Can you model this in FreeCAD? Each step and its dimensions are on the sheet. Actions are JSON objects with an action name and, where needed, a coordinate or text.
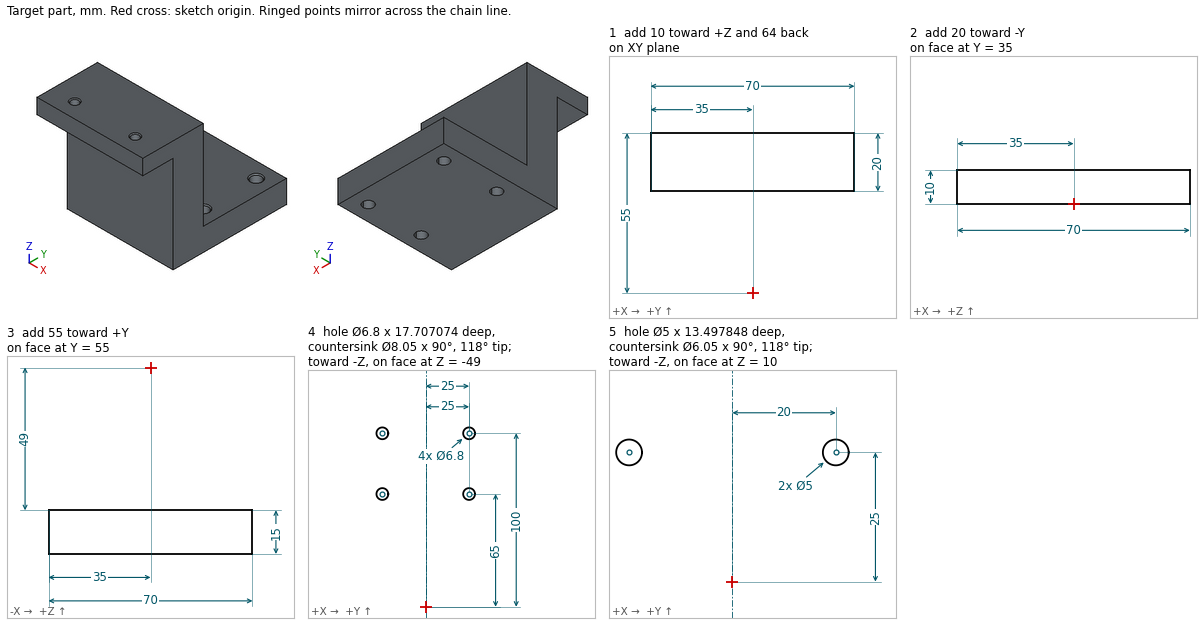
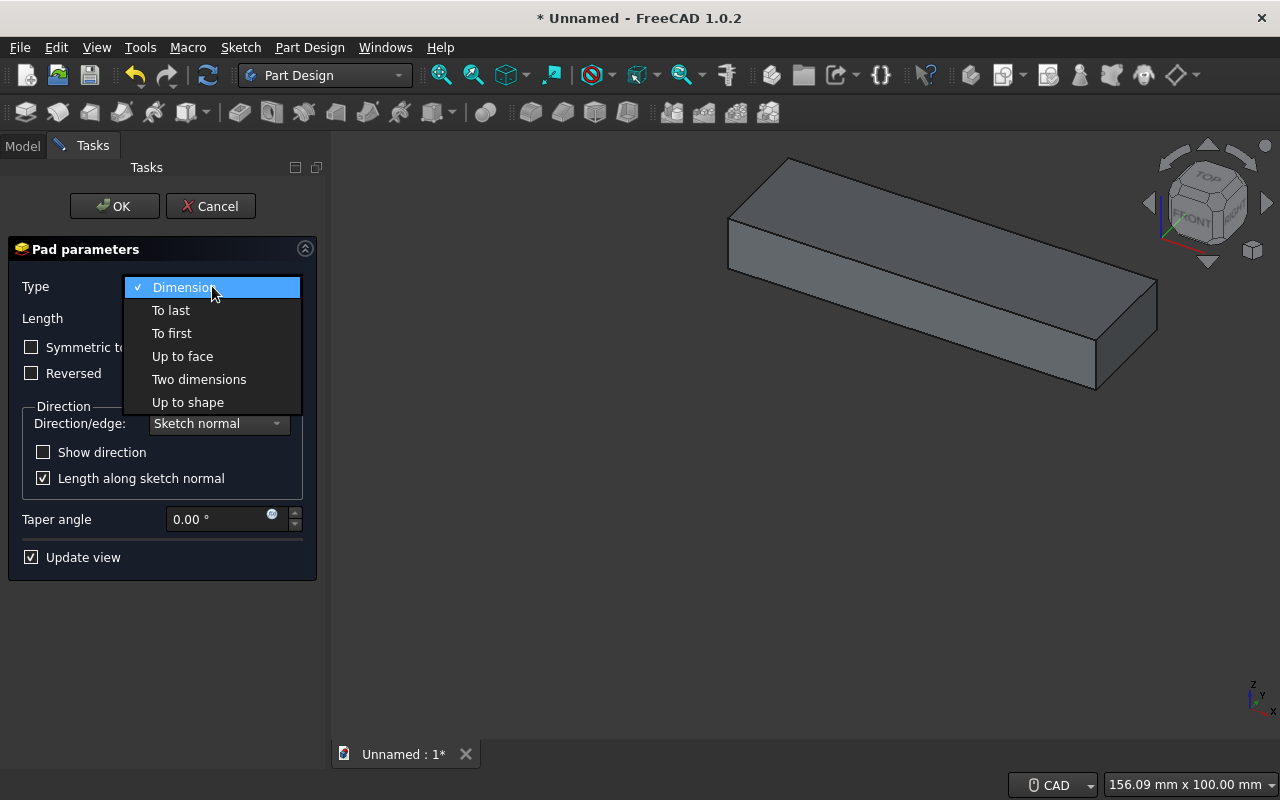
{"action": "left_click", "coordinate": [212, 380]}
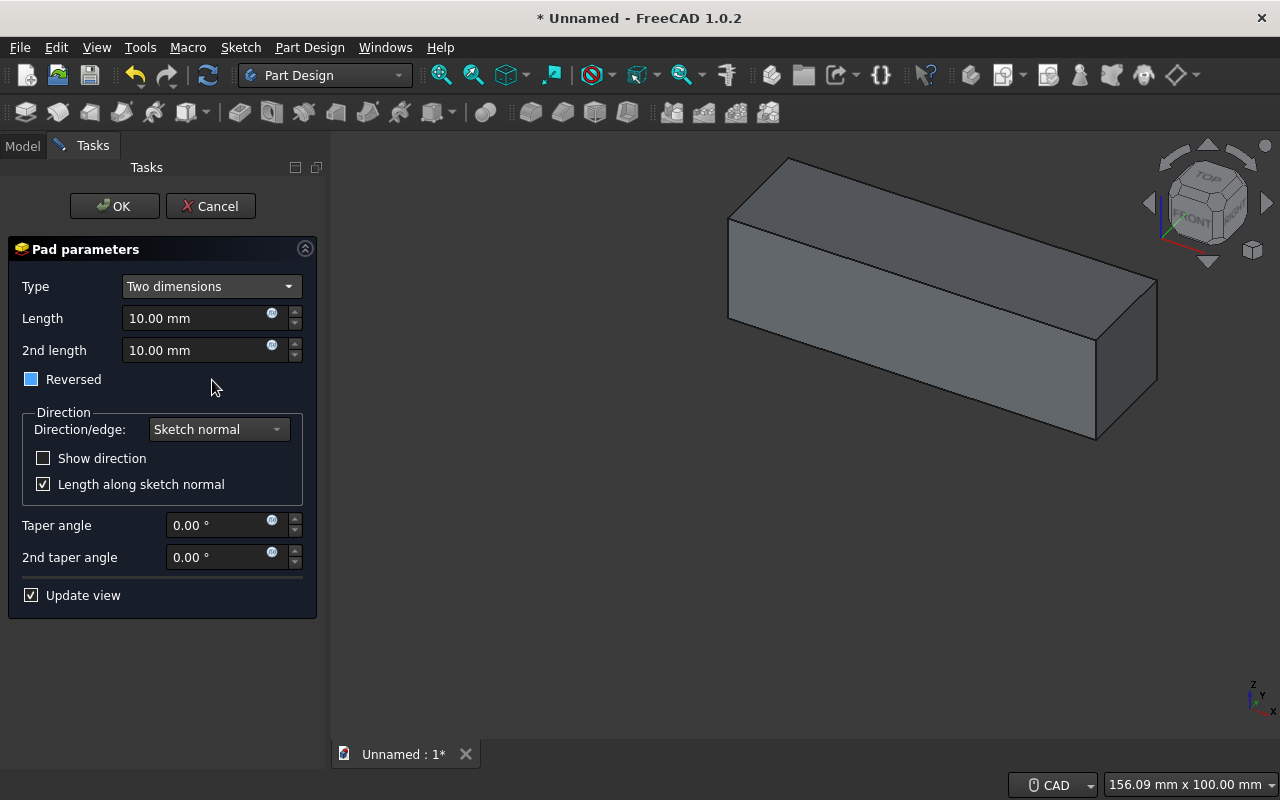
{"action": "triple_click", "coordinate": [204, 318]}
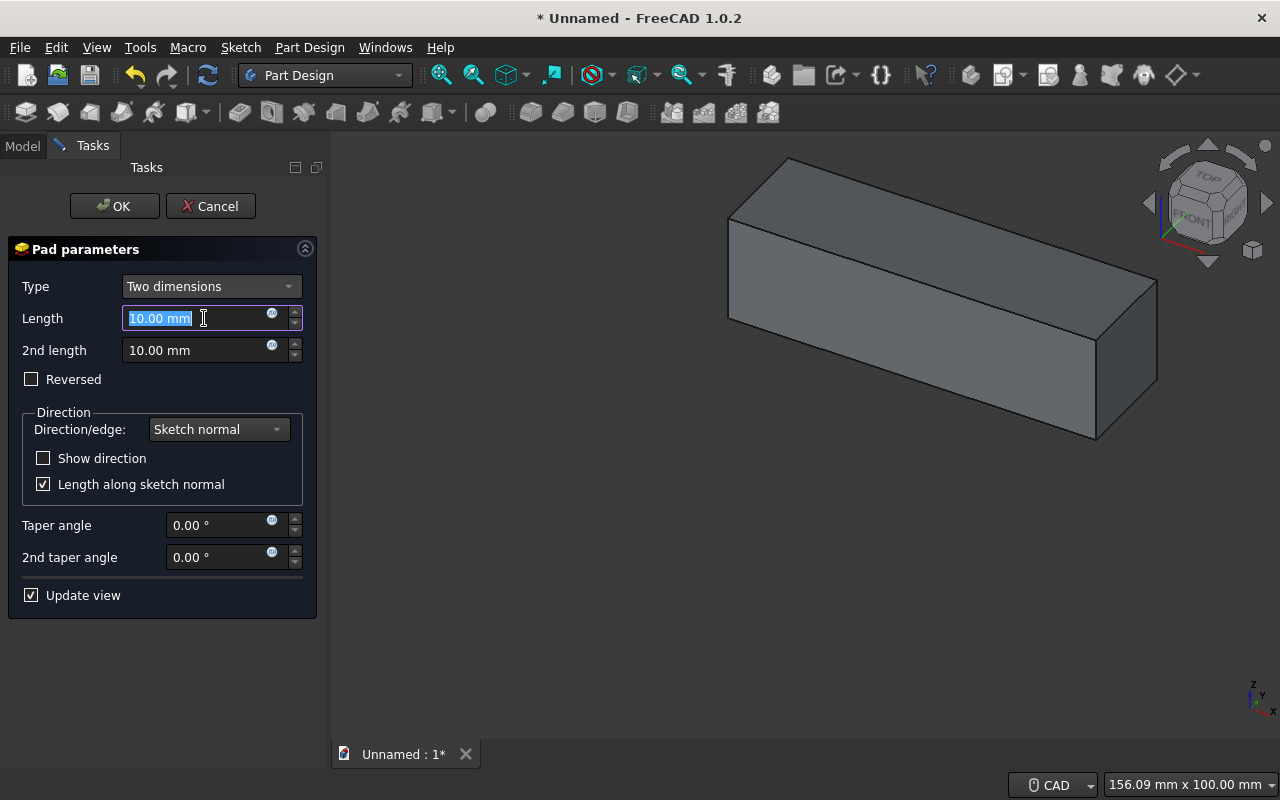
{"action": "type", "text": "10"}
{"action": "key", "text": "Tab"}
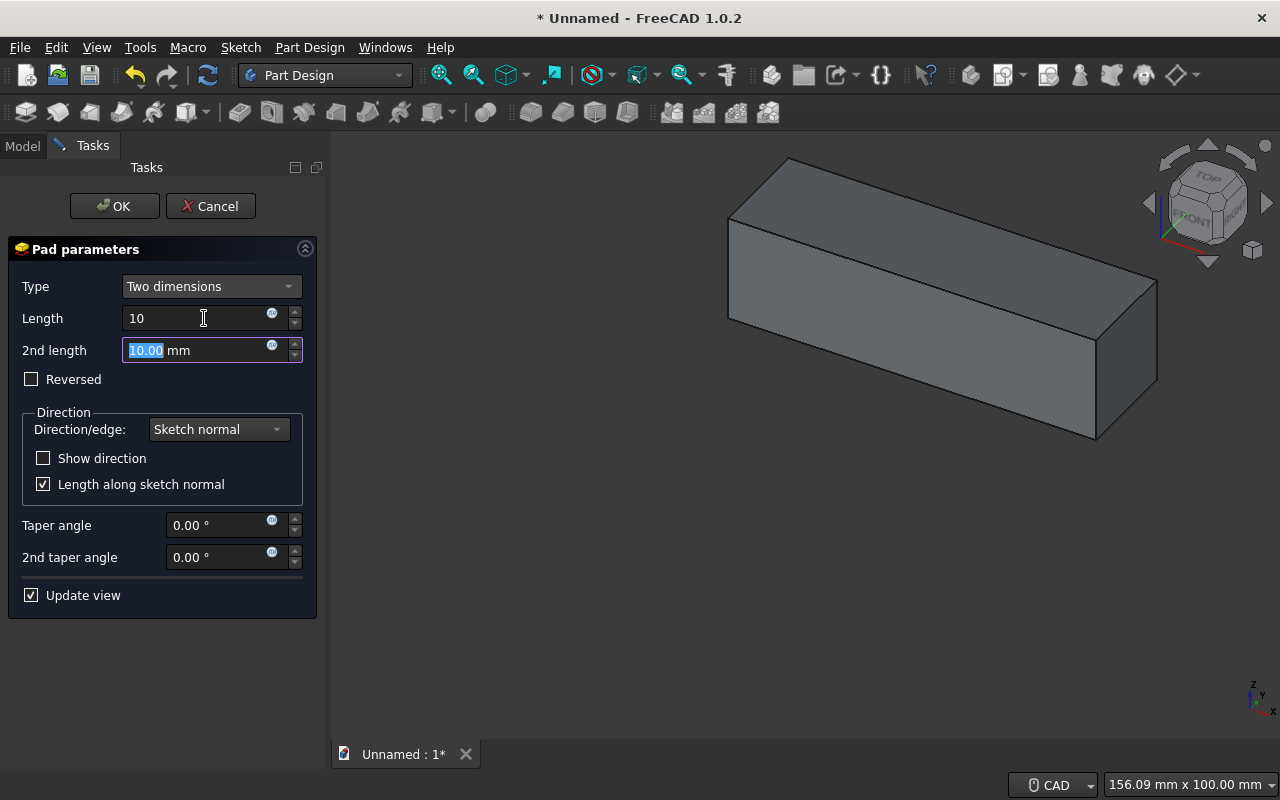
{"action": "type", "text": "64"}
{"action": "key", "text": "Tab"}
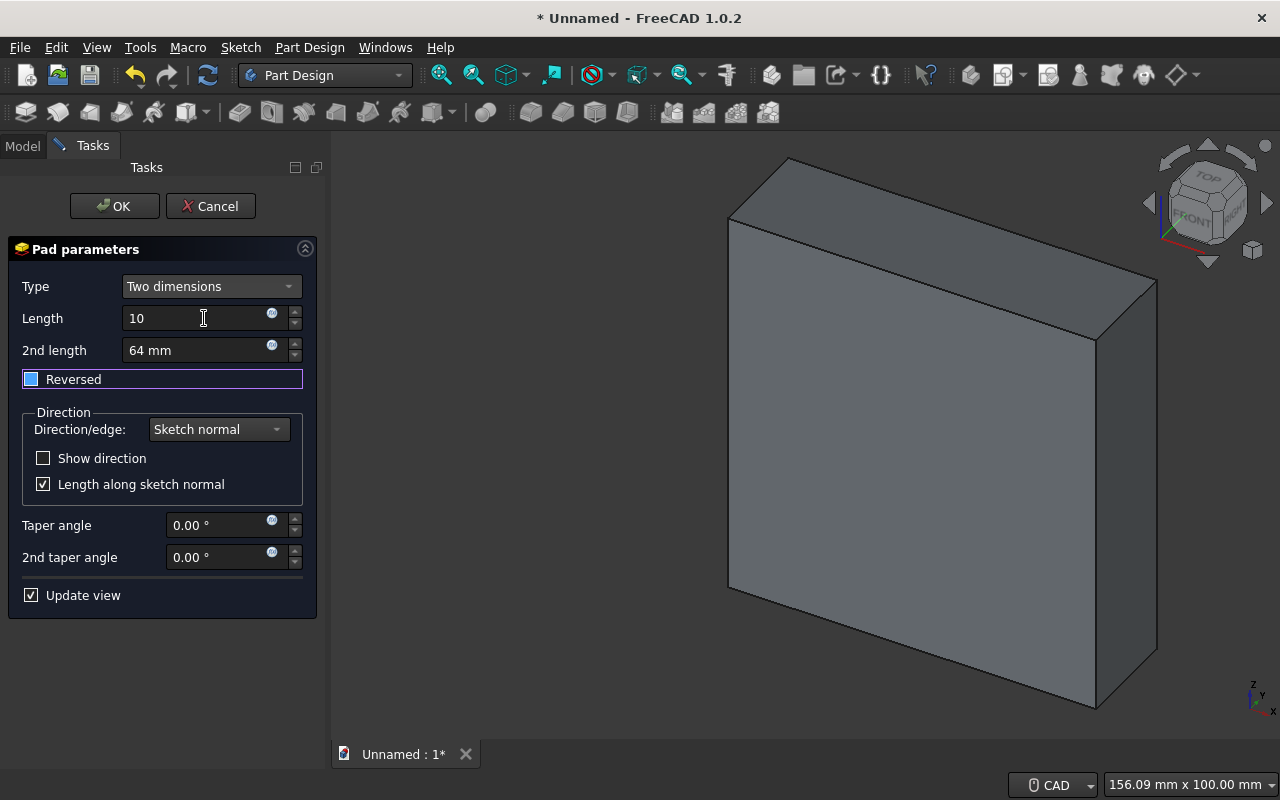
{"action": "left_click", "coordinate": [115, 206]}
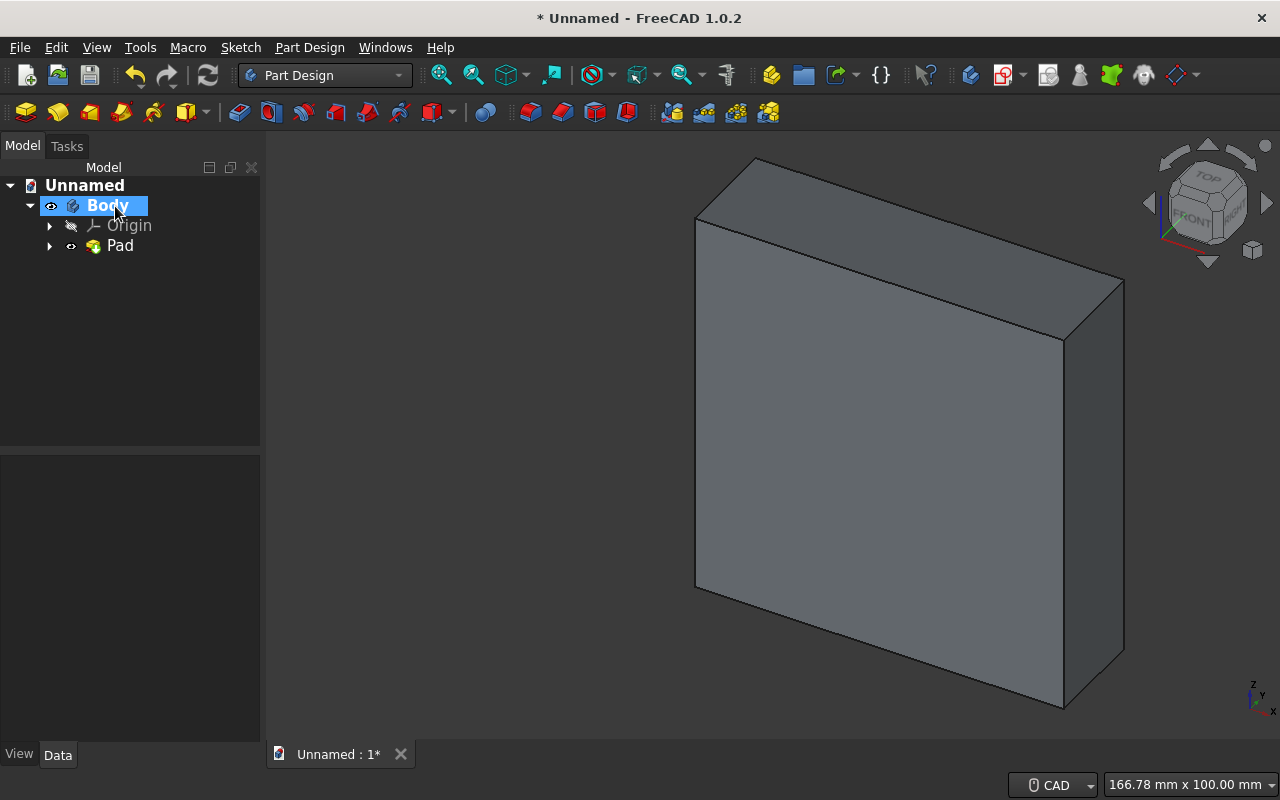
{"action": "left_click", "coordinate": [879, 463]}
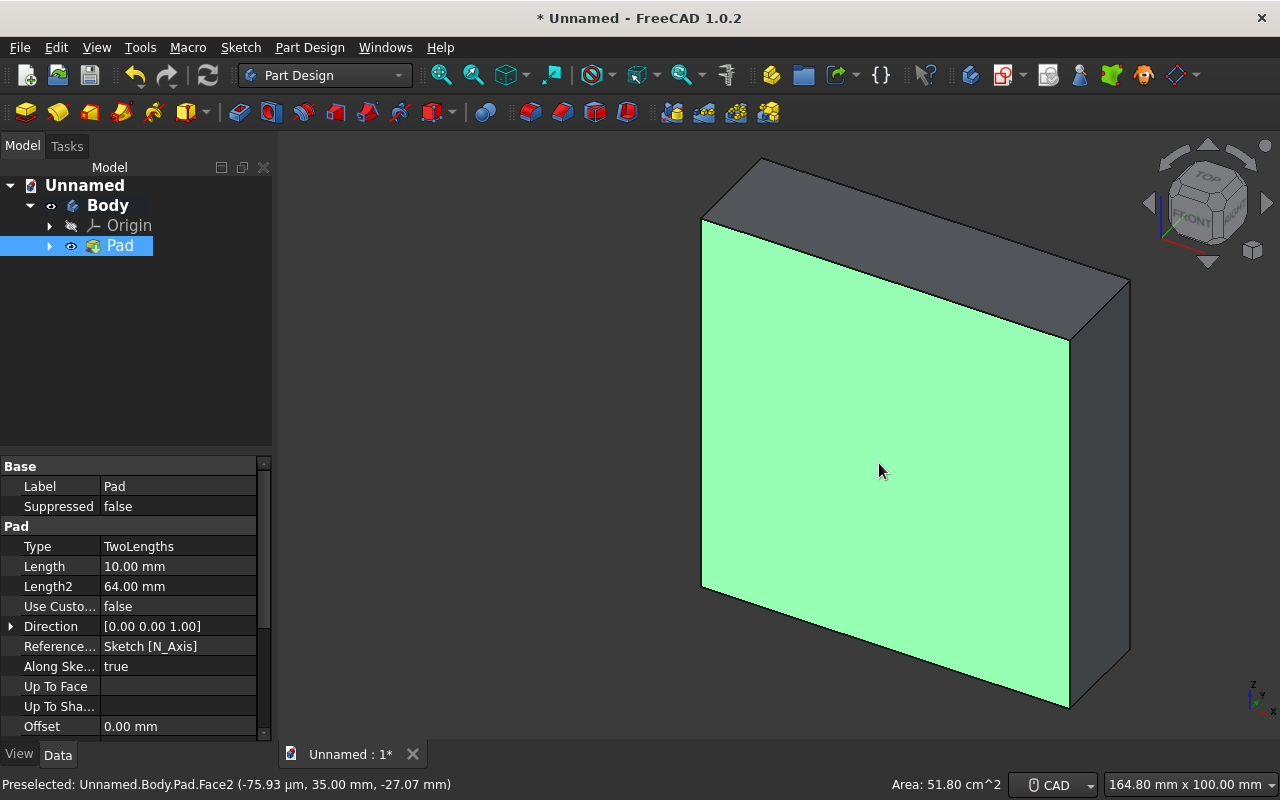
{"action": "left_click", "coordinate": [1004, 76]}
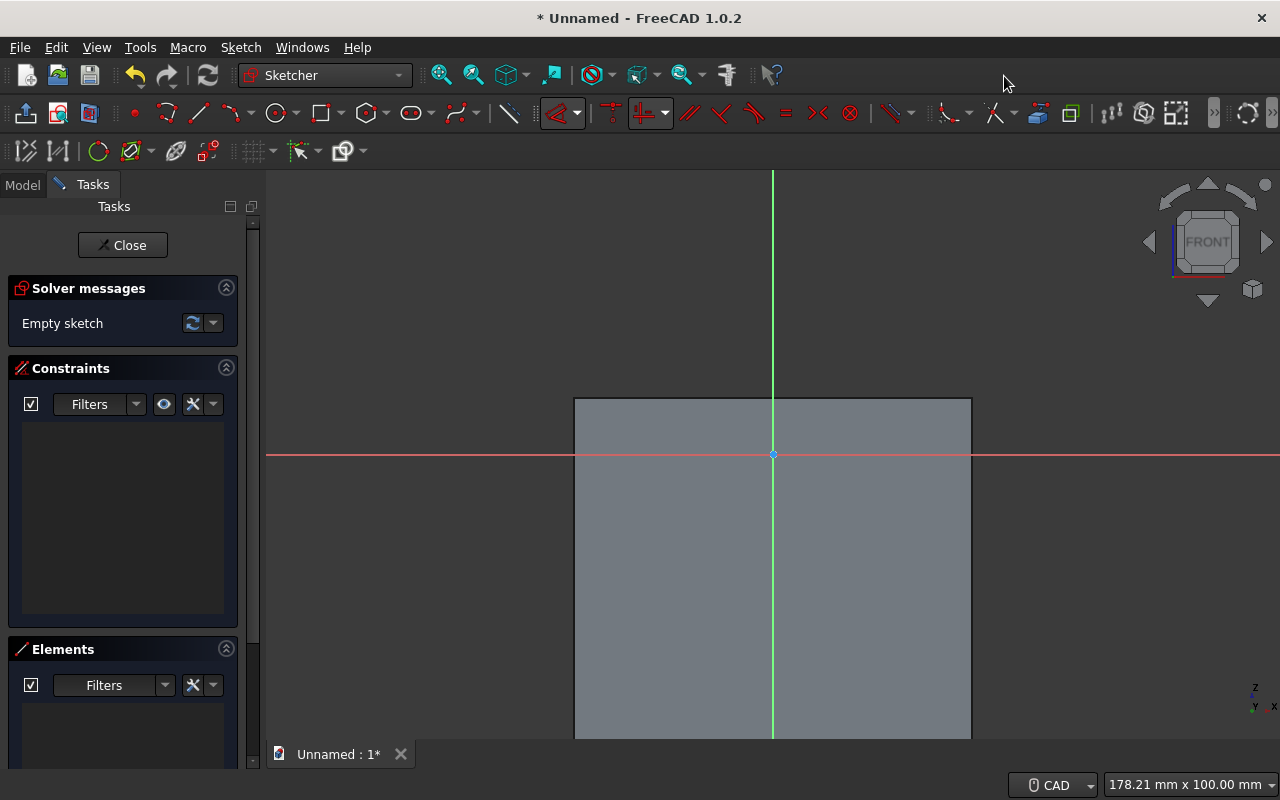
{"action": "scroll", "coordinate": [912, 368], "scroll_direction": "up", "scroll_amount": 2}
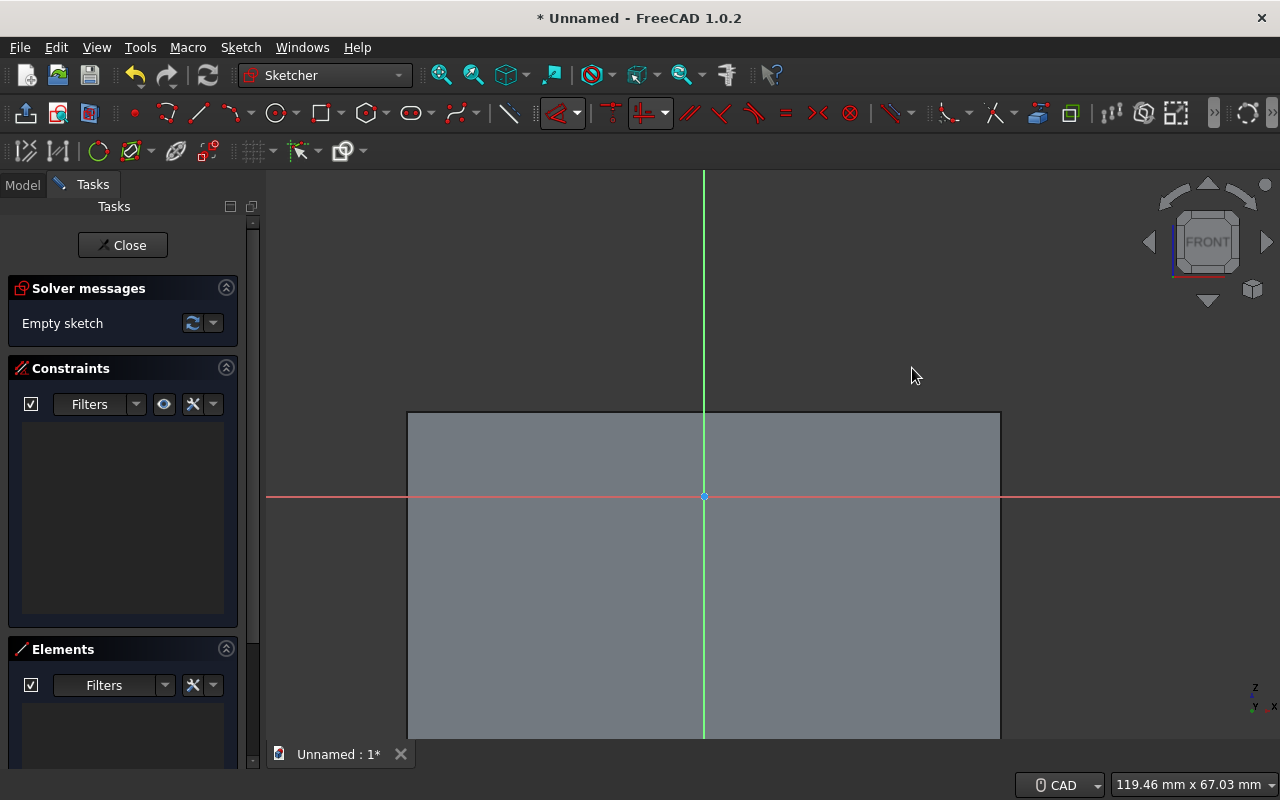
{"action": "left_click", "coordinate": [322, 114]}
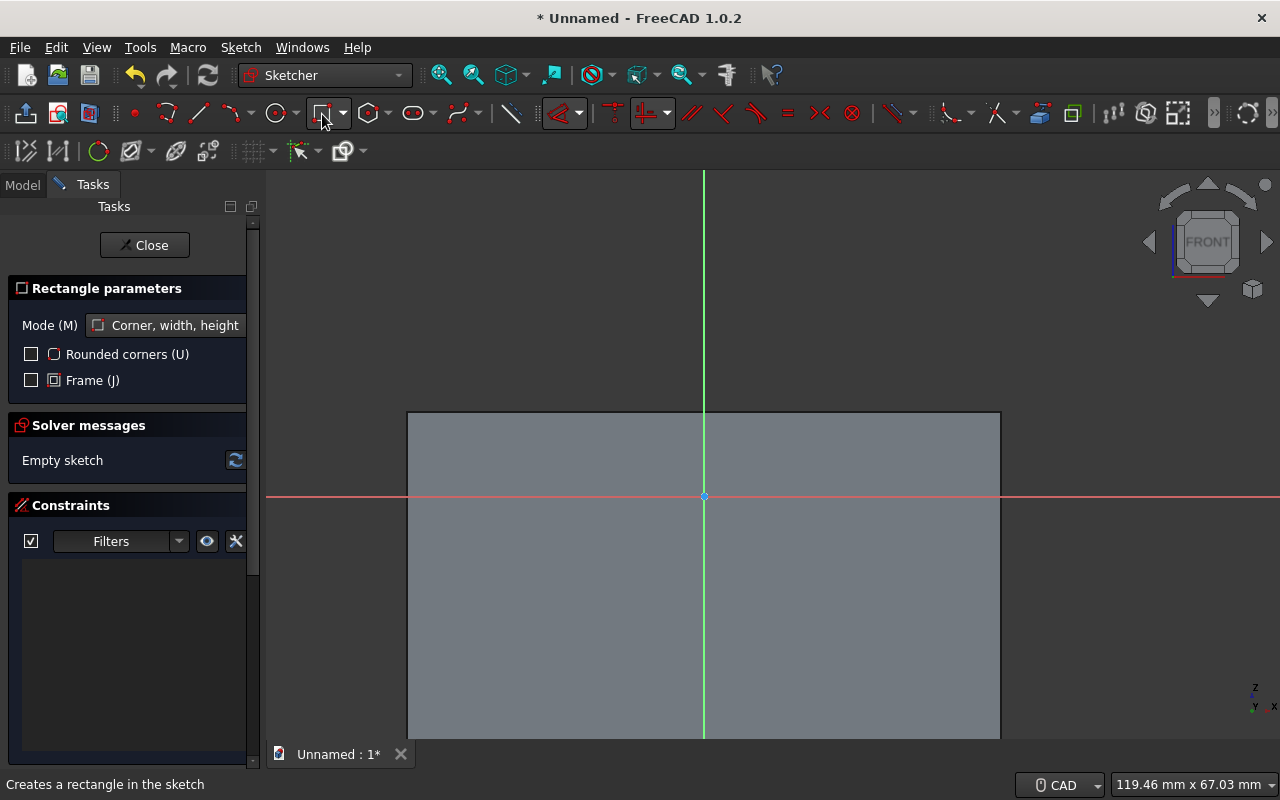
{"action": "left_click", "coordinate": [407, 412]}
{"action": "left_click", "coordinate": [1001, 497]}
{"action": "key", "text": "Escape"}